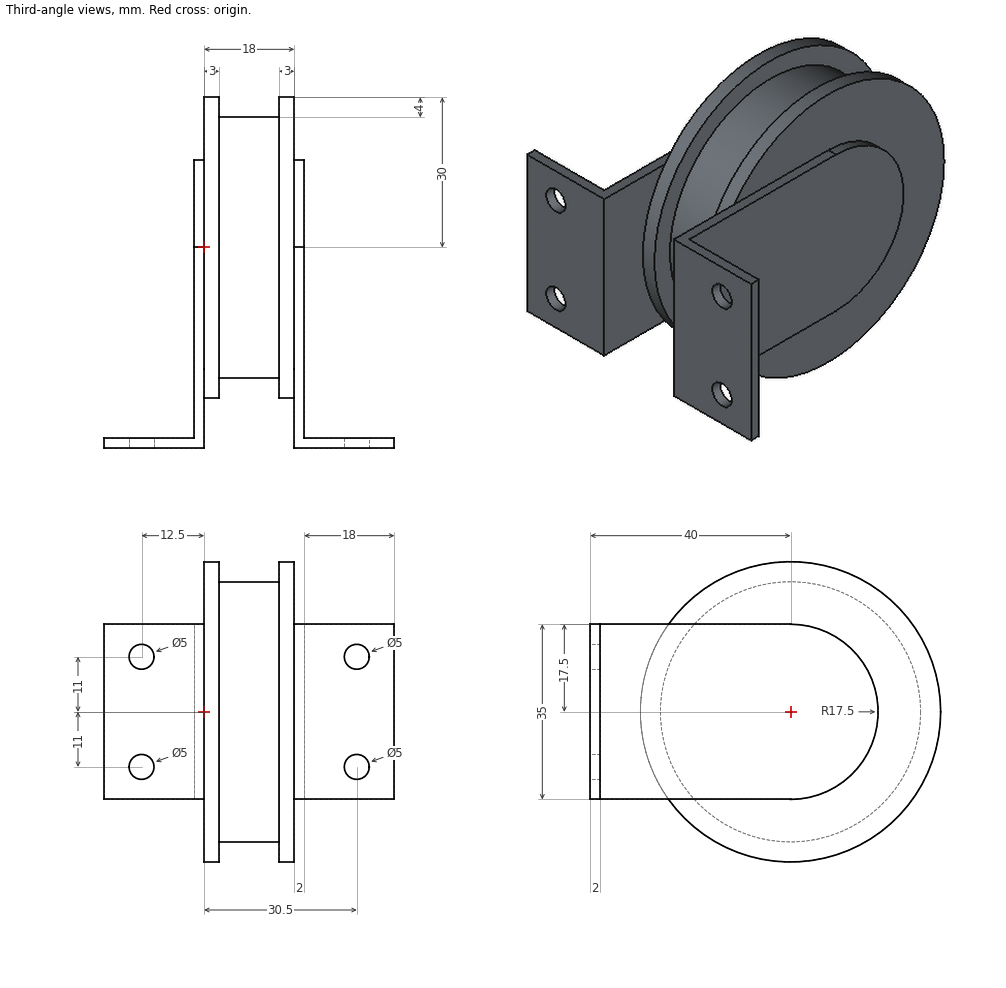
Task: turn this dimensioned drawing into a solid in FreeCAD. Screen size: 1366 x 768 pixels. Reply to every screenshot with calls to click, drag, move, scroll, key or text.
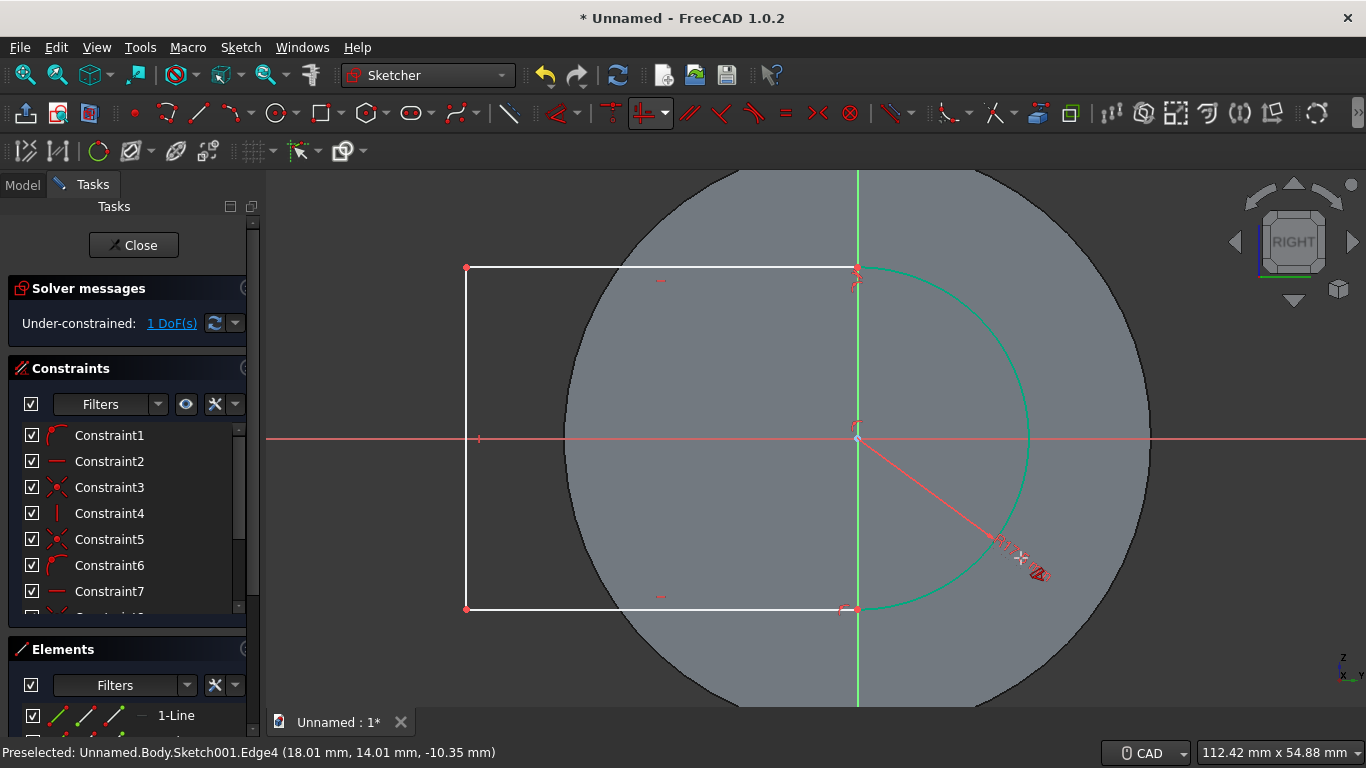
click(740, 267)
click(662, 233)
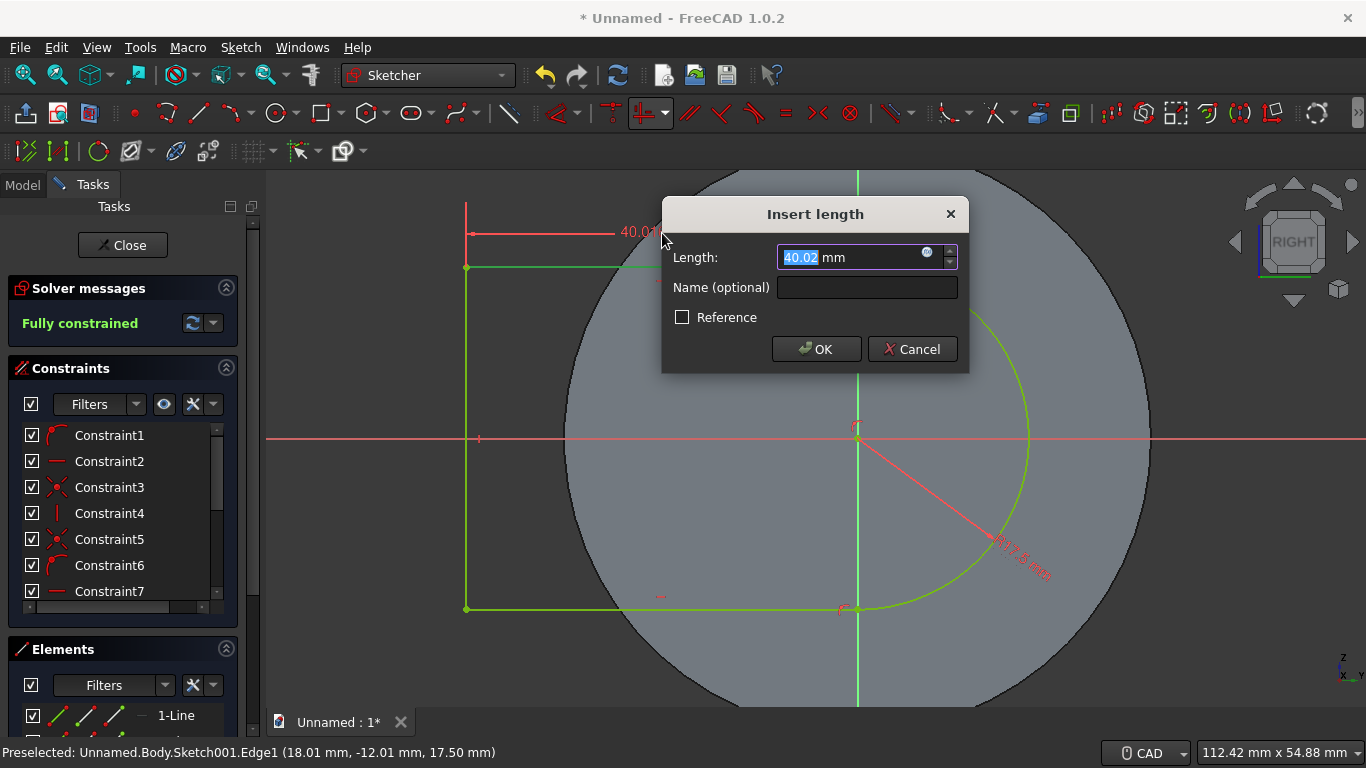
text(40)
key(Return)
key(Escape)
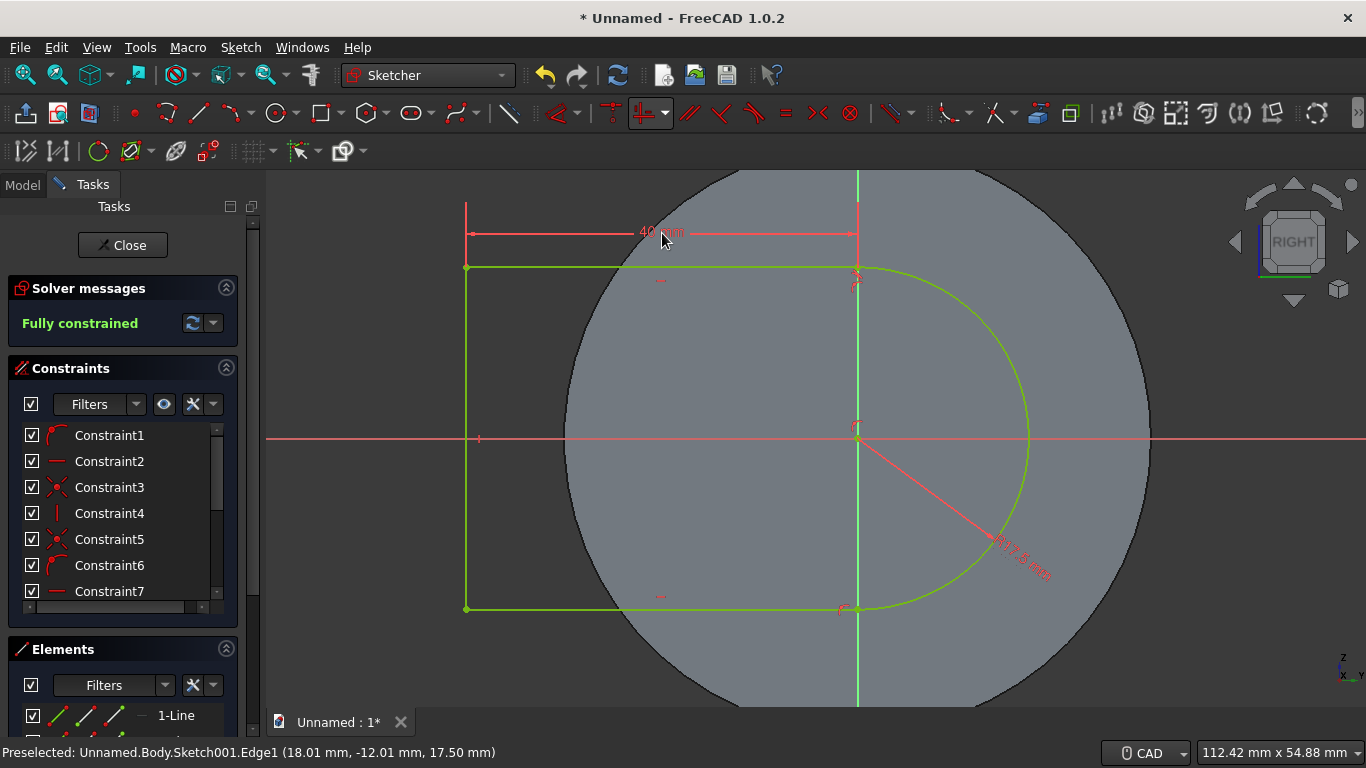
click(123, 245)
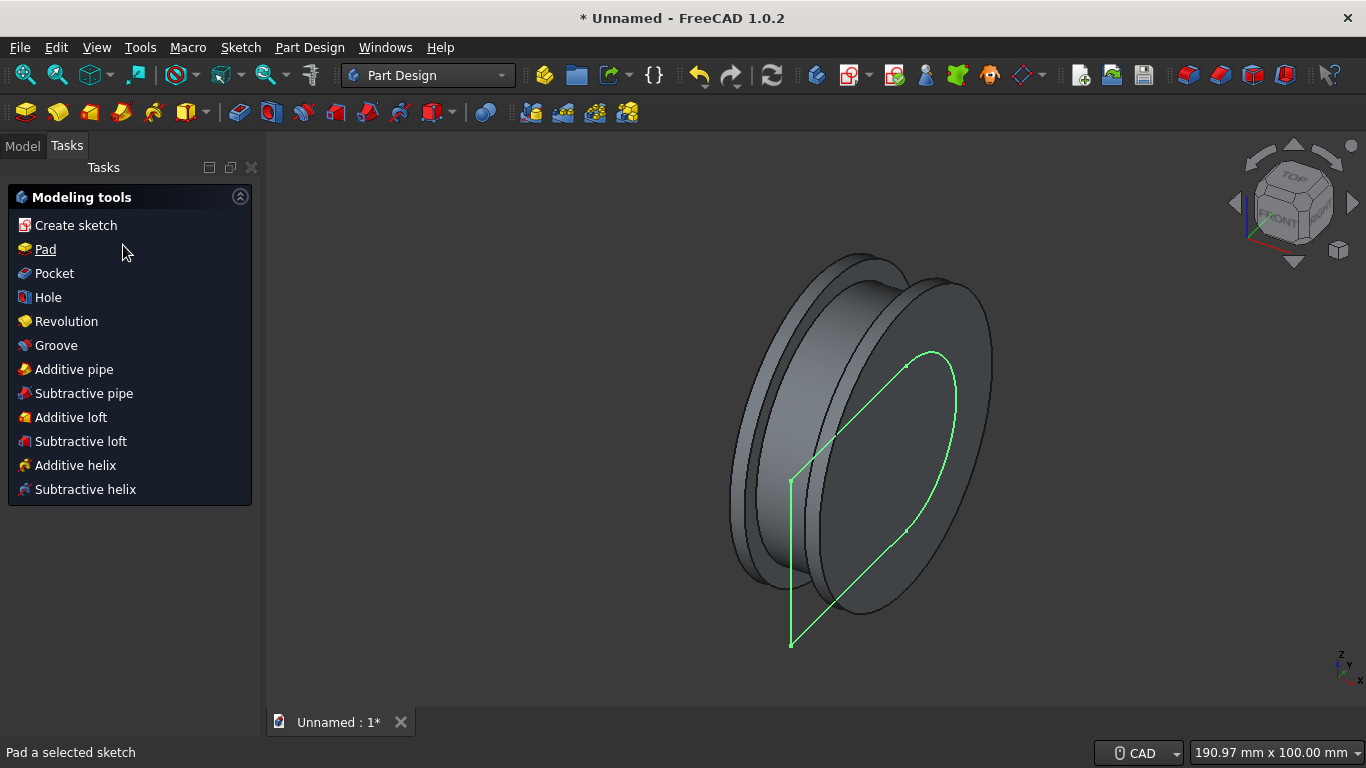
click(26, 112)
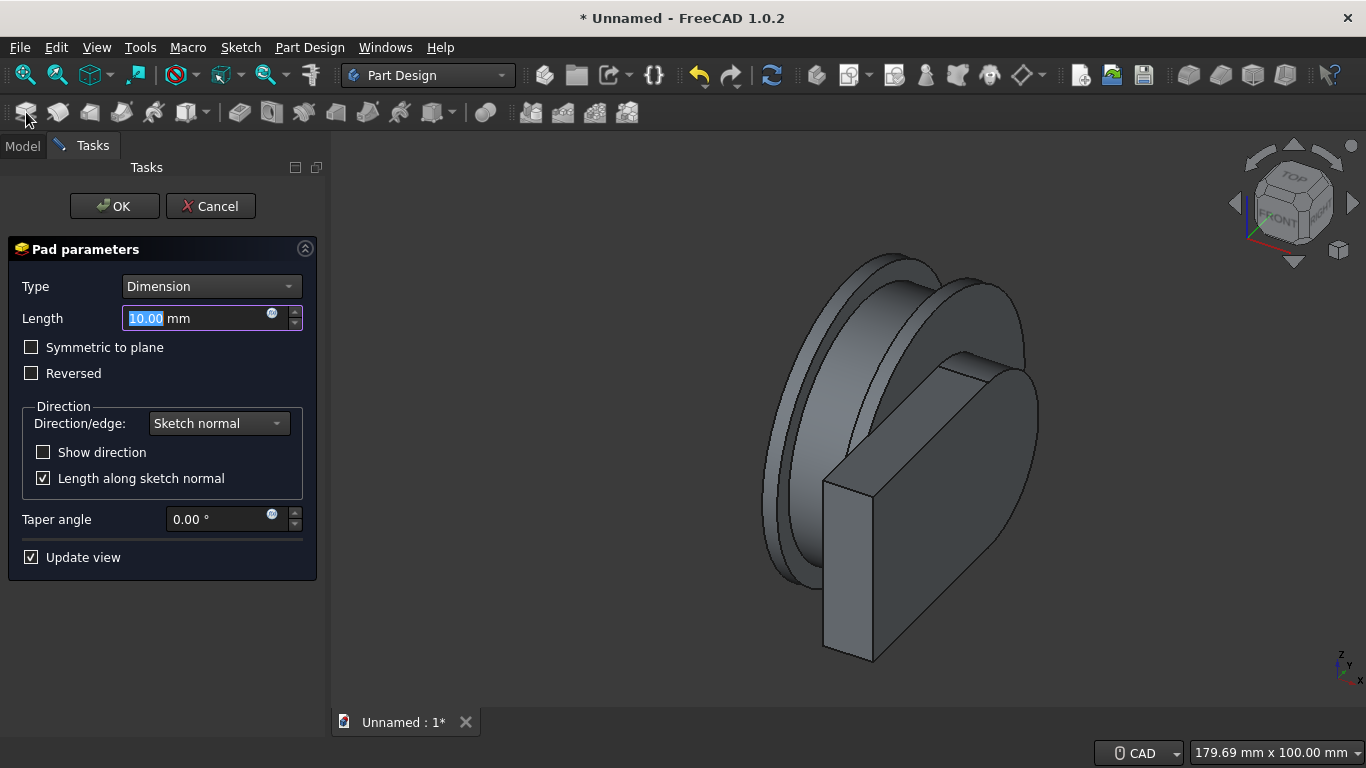
text(2)
key(Tab)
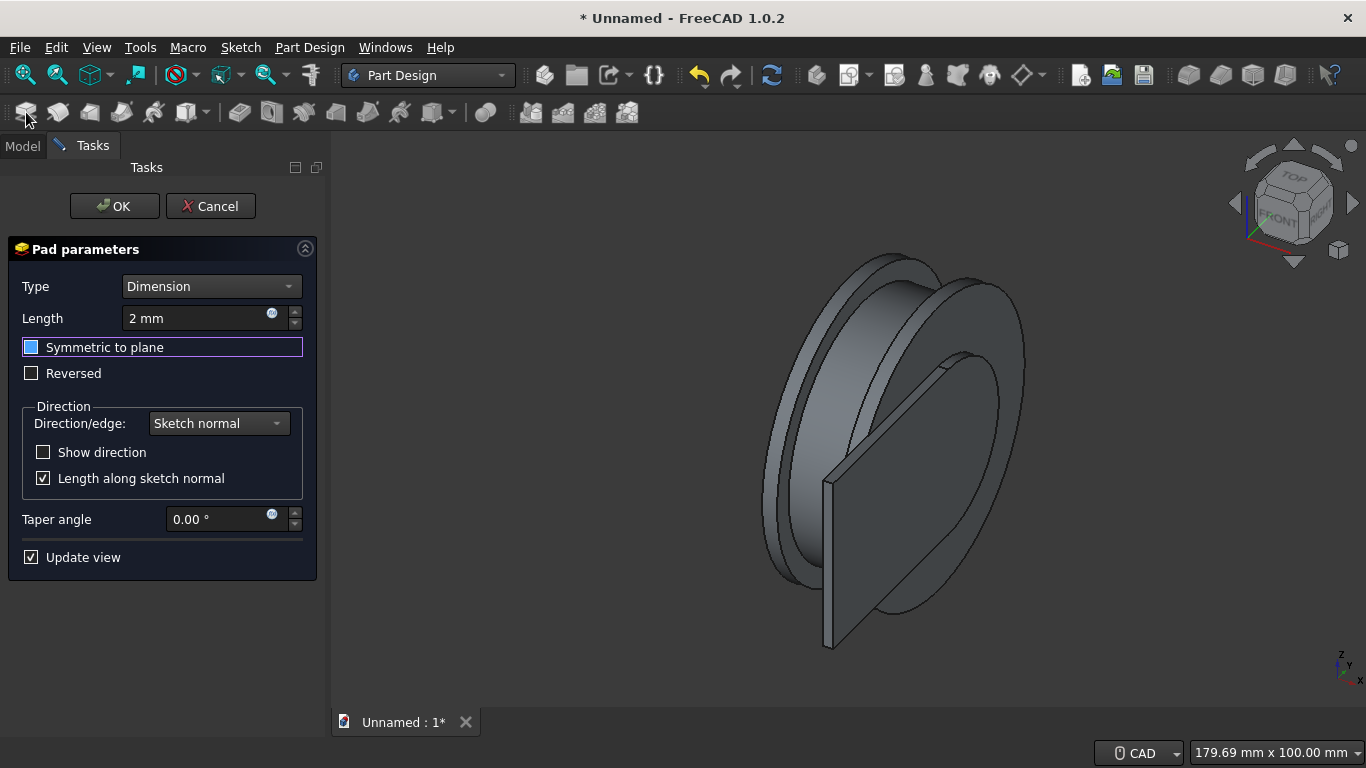
click(115, 206)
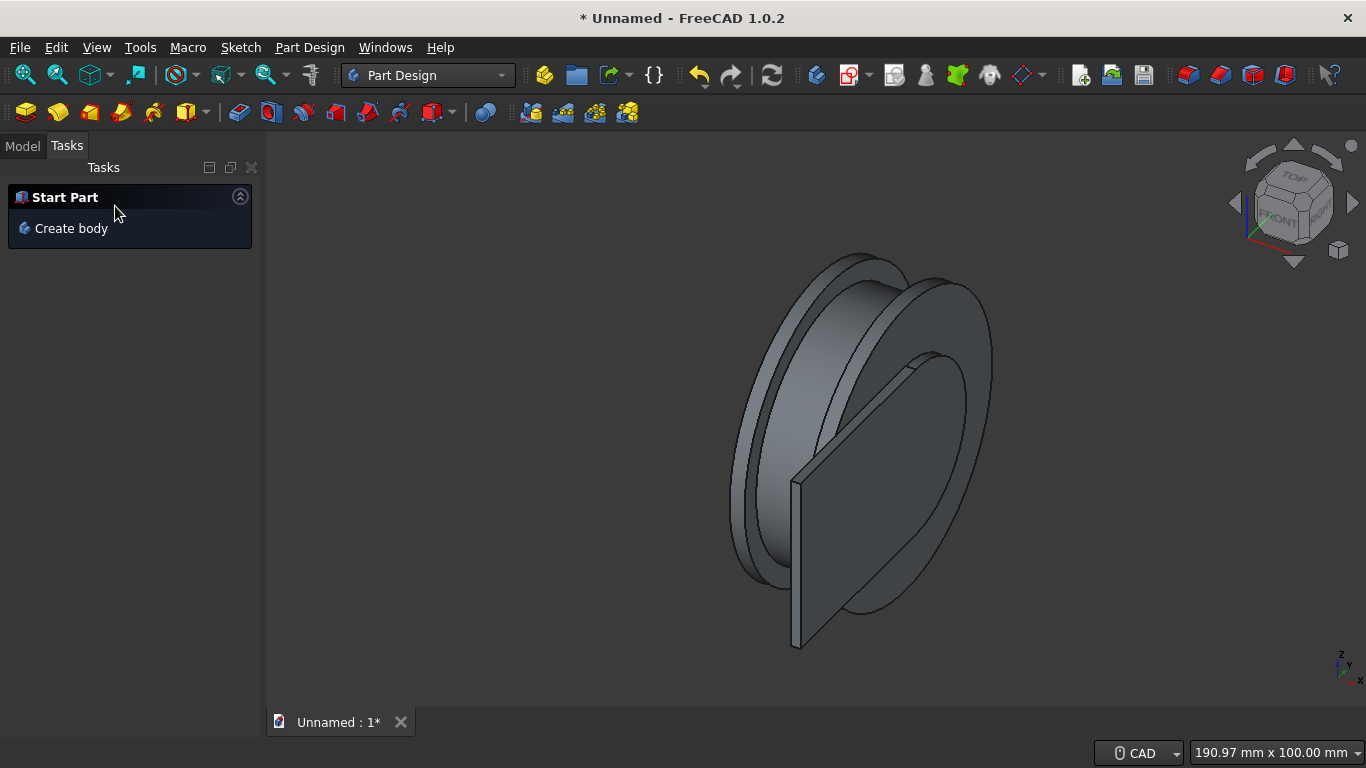
click(907, 460)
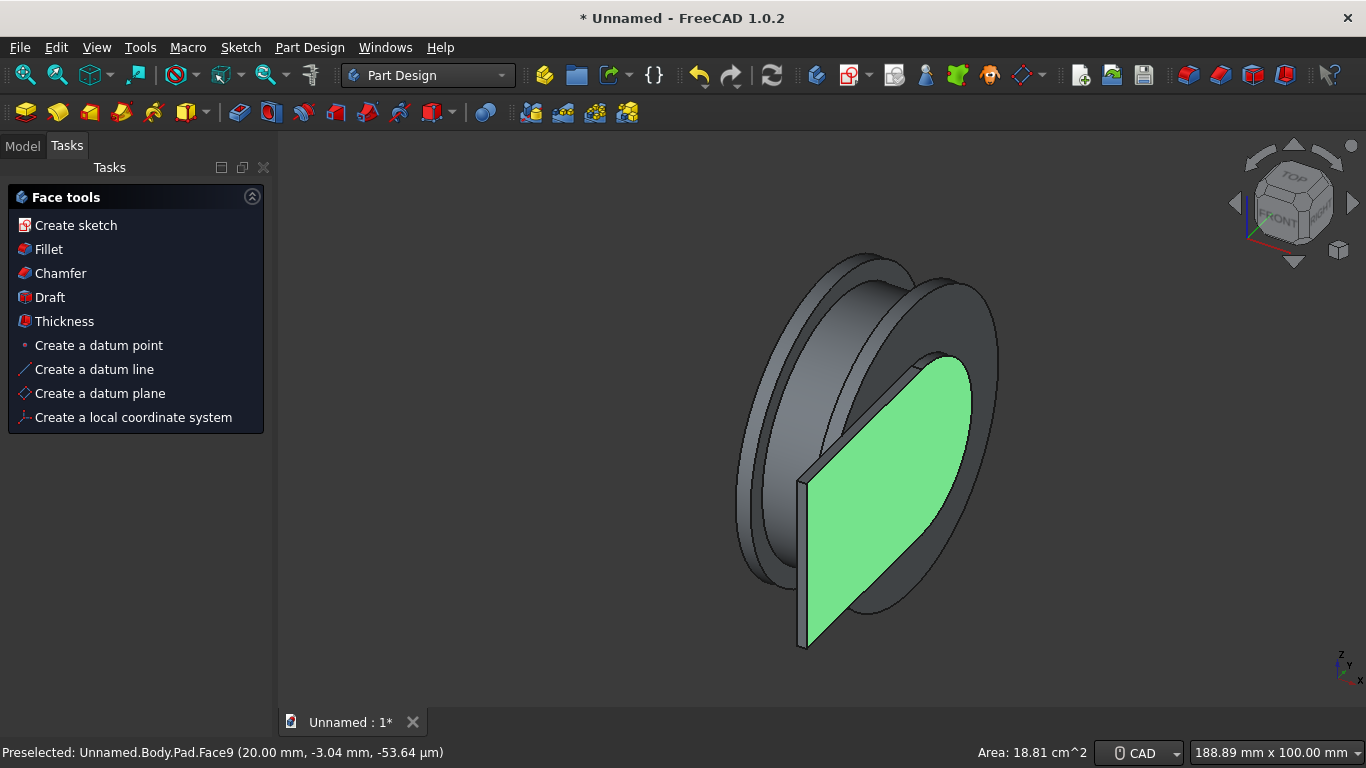
click(850, 76)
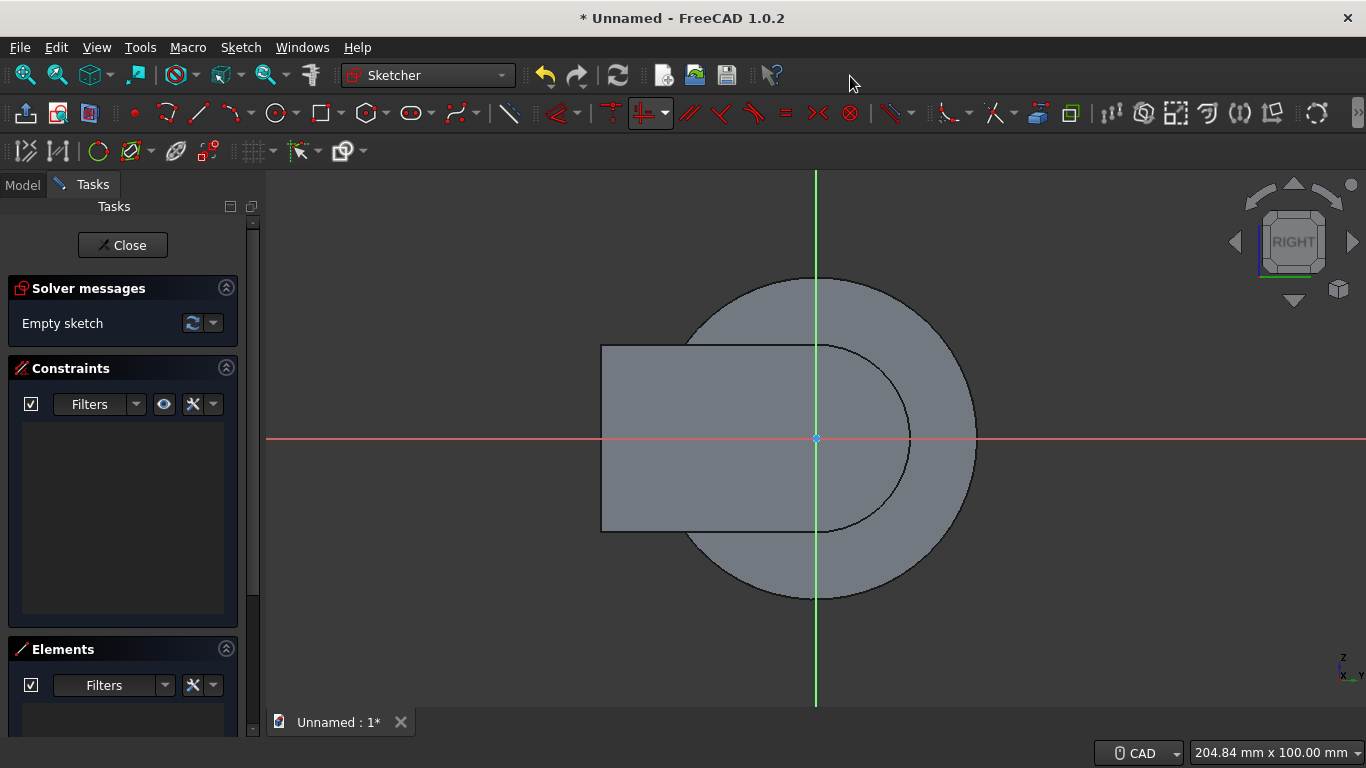
scroll(661, 438, up, 3)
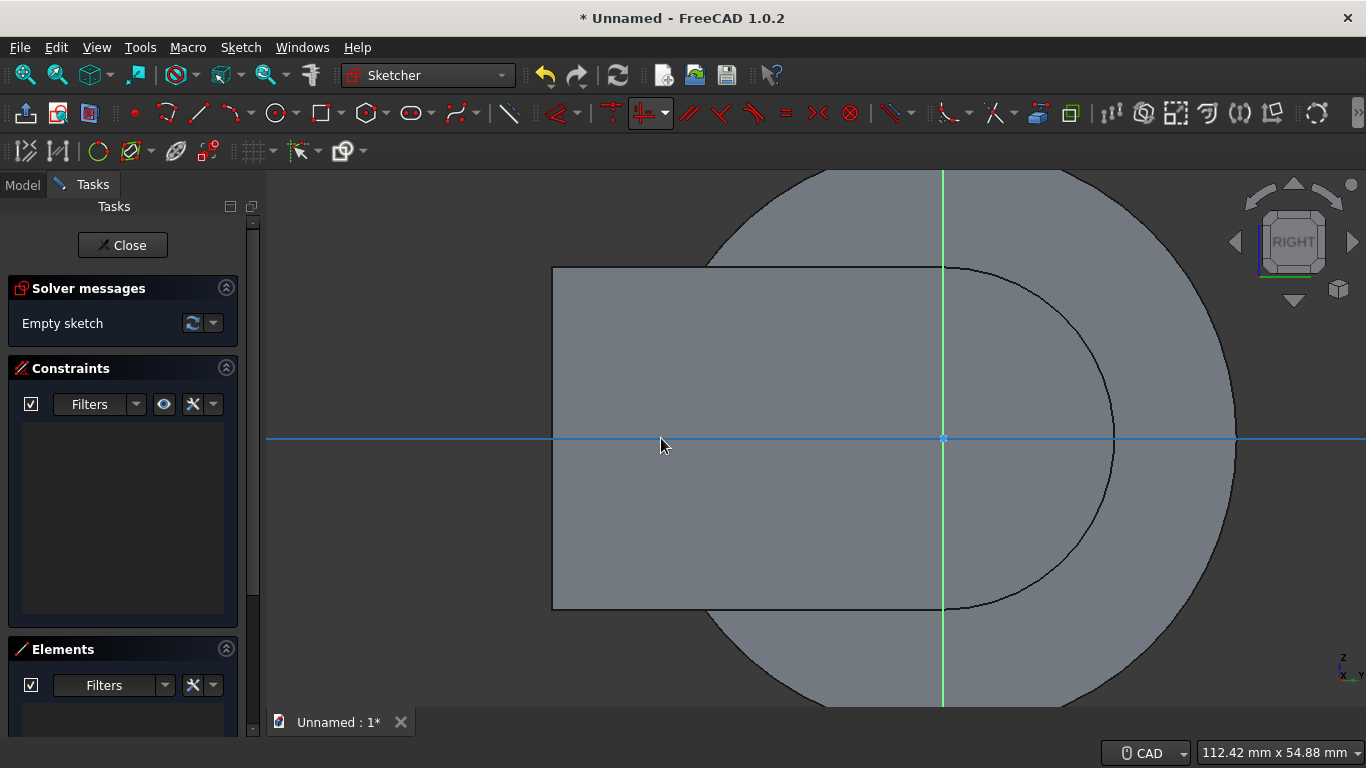
click(322, 114)